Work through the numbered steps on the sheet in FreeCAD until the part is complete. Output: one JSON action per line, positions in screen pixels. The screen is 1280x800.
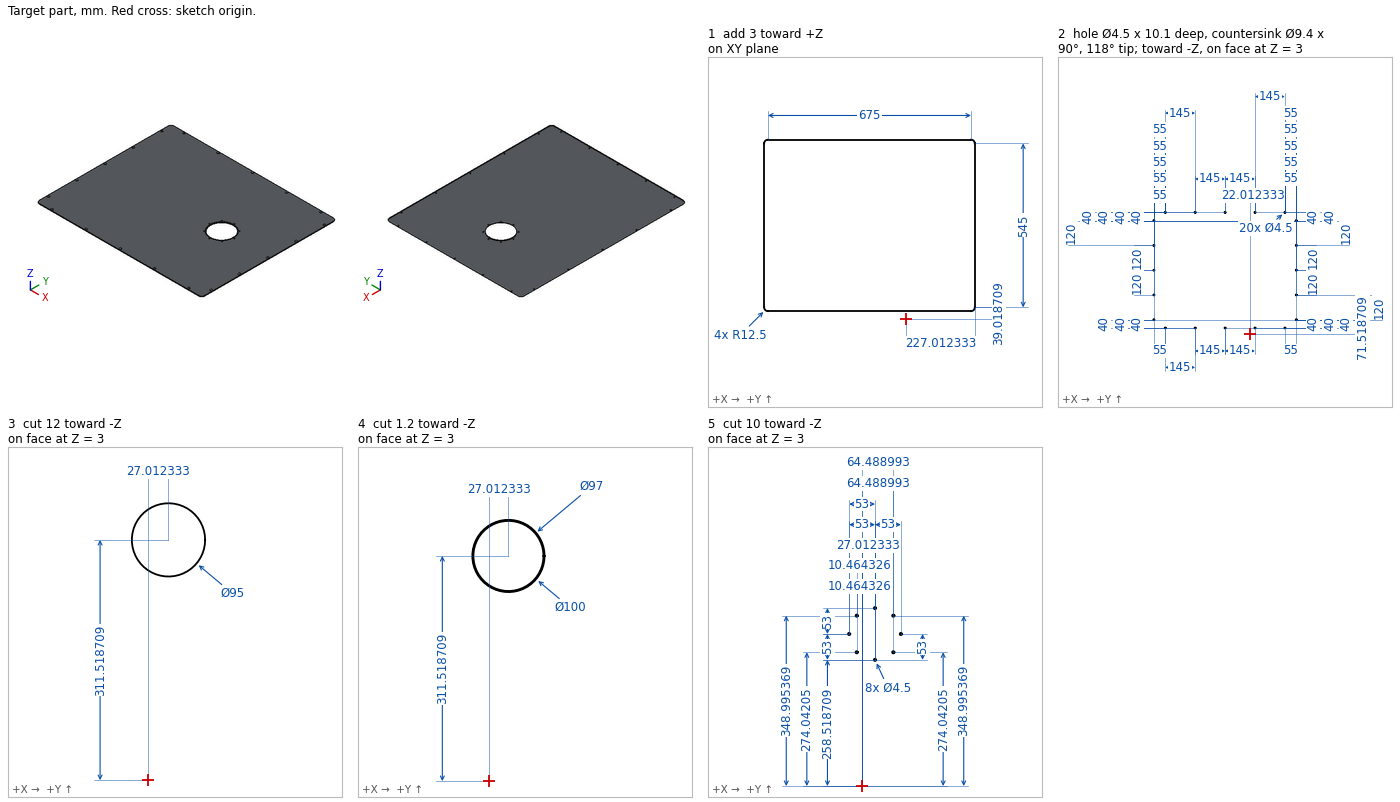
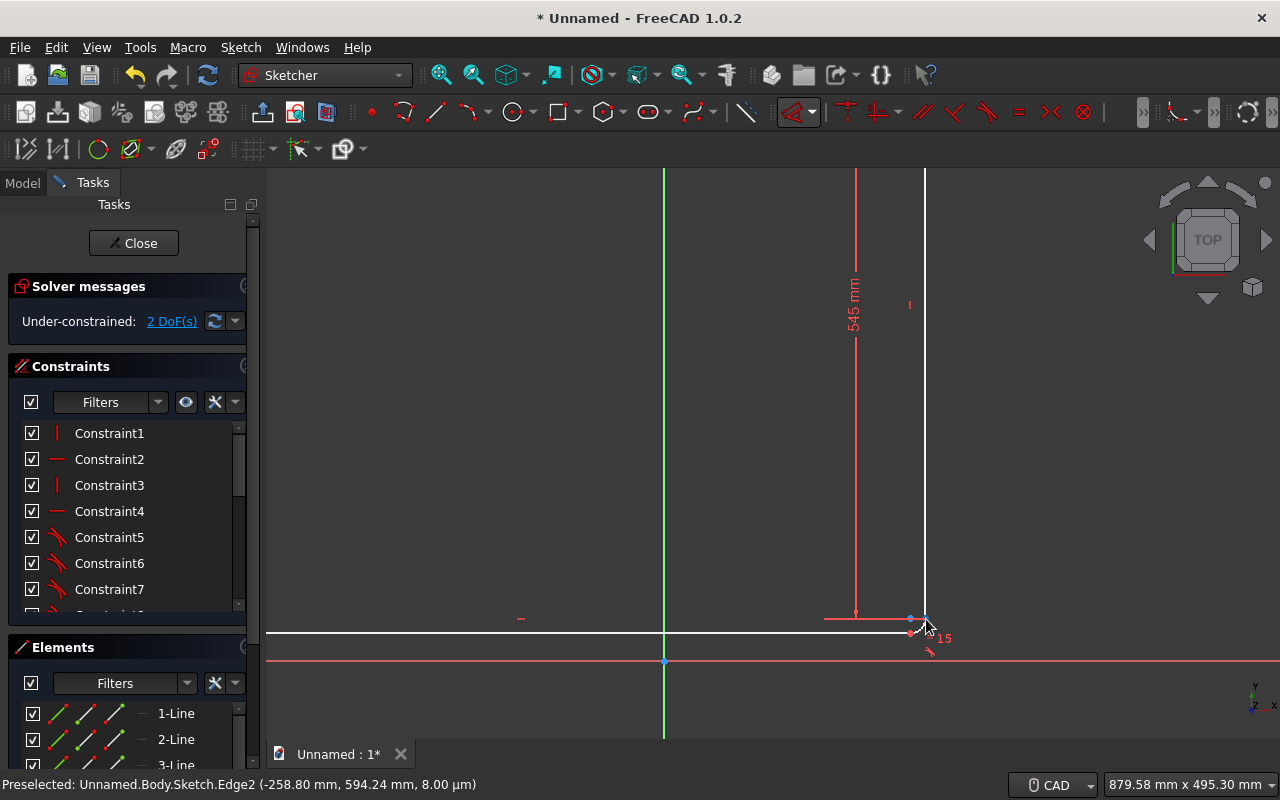
{"action": "left_click", "coordinate": [925, 619]}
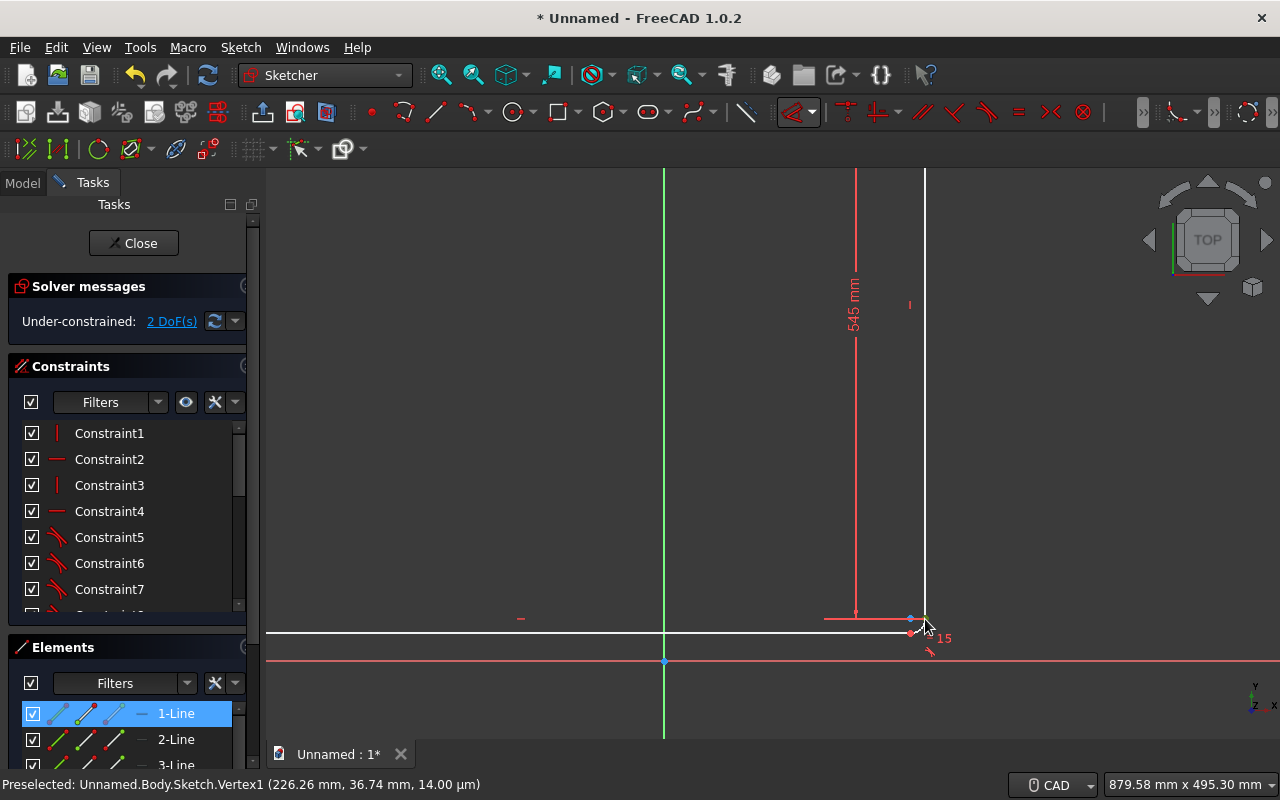
{"action": "left_click", "coordinate": [814, 112]}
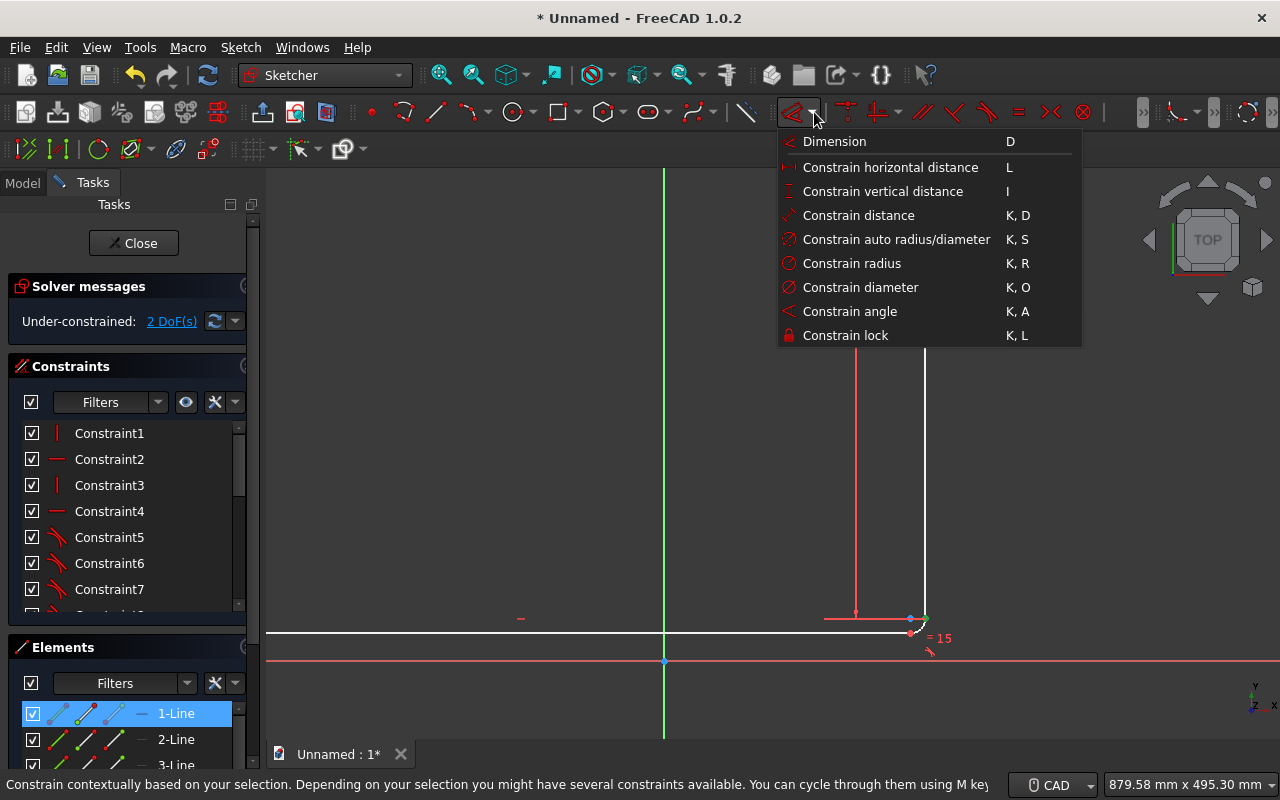
{"action": "left_click", "coordinate": [930, 191]}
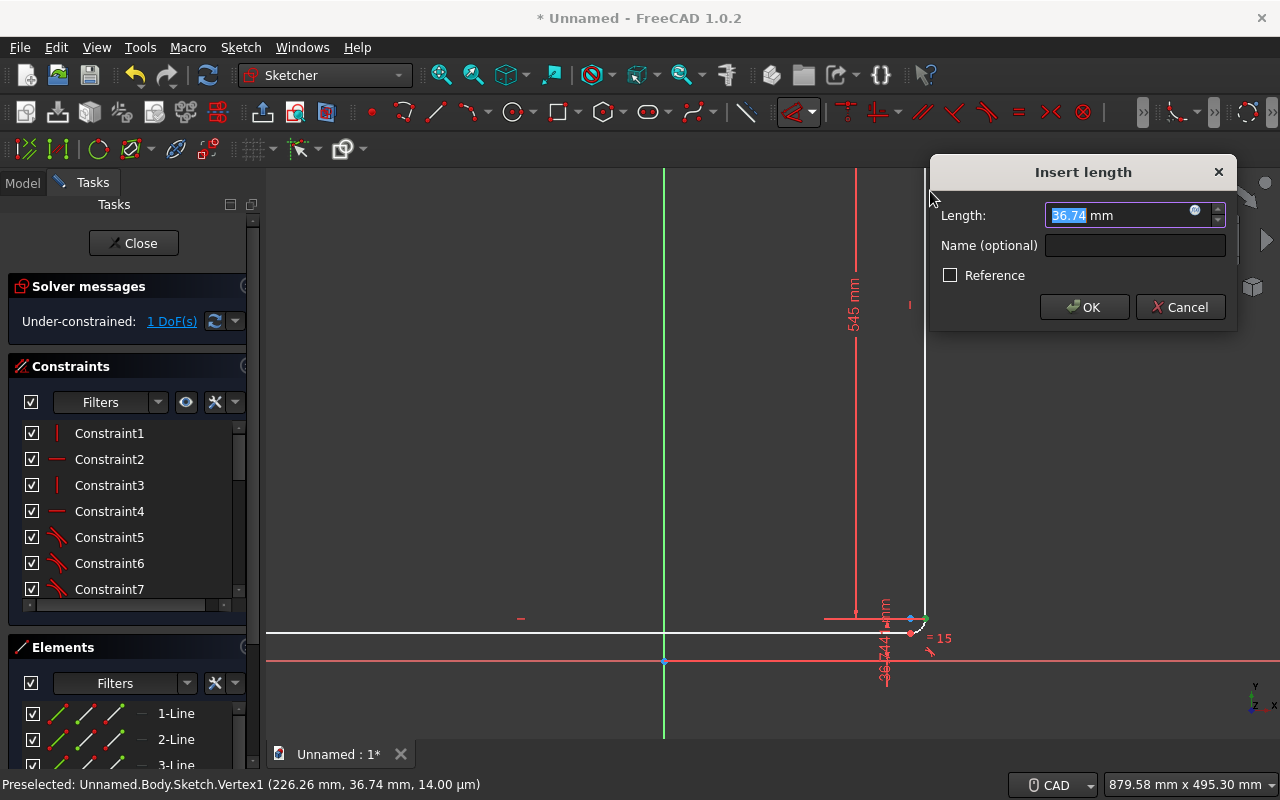
{"action": "type", "text": "39.018709"}
{"action": "key", "text": "Return"}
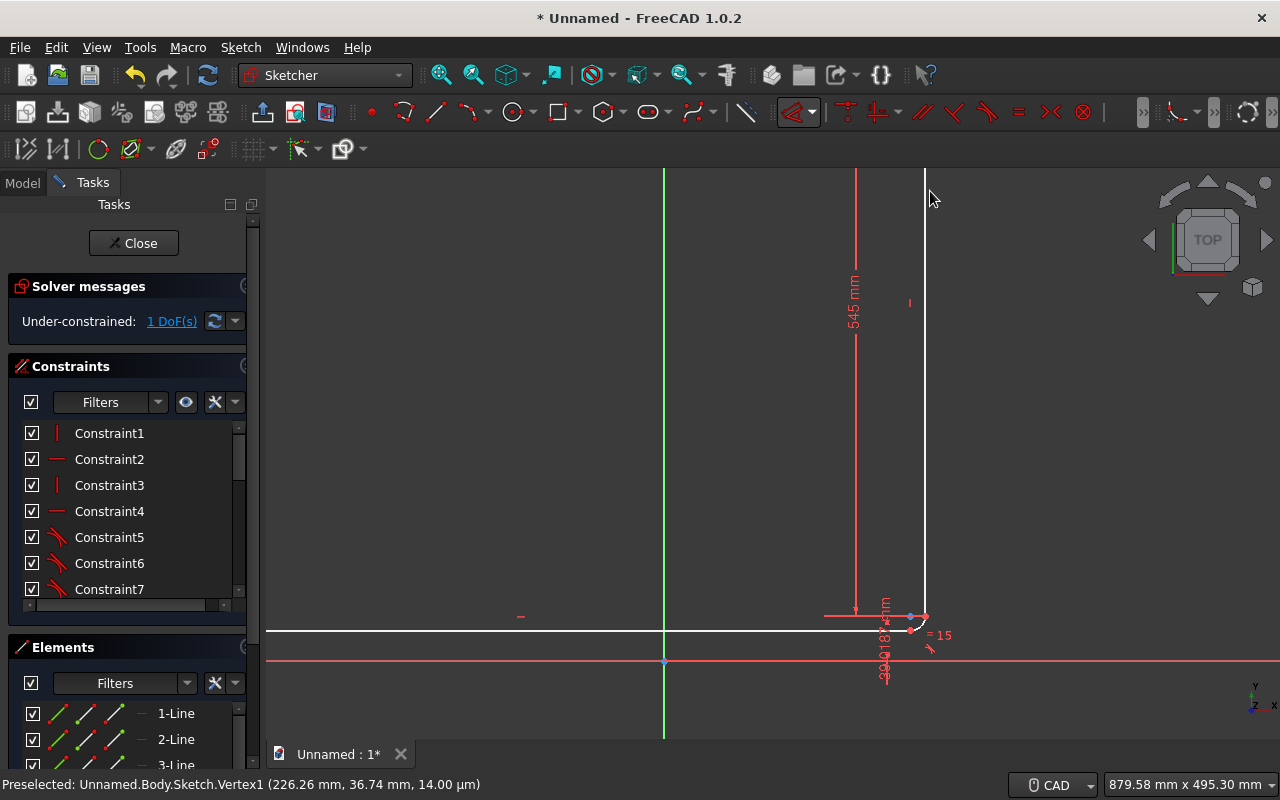
{"action": "left_click", "coordinate": [925, 616]}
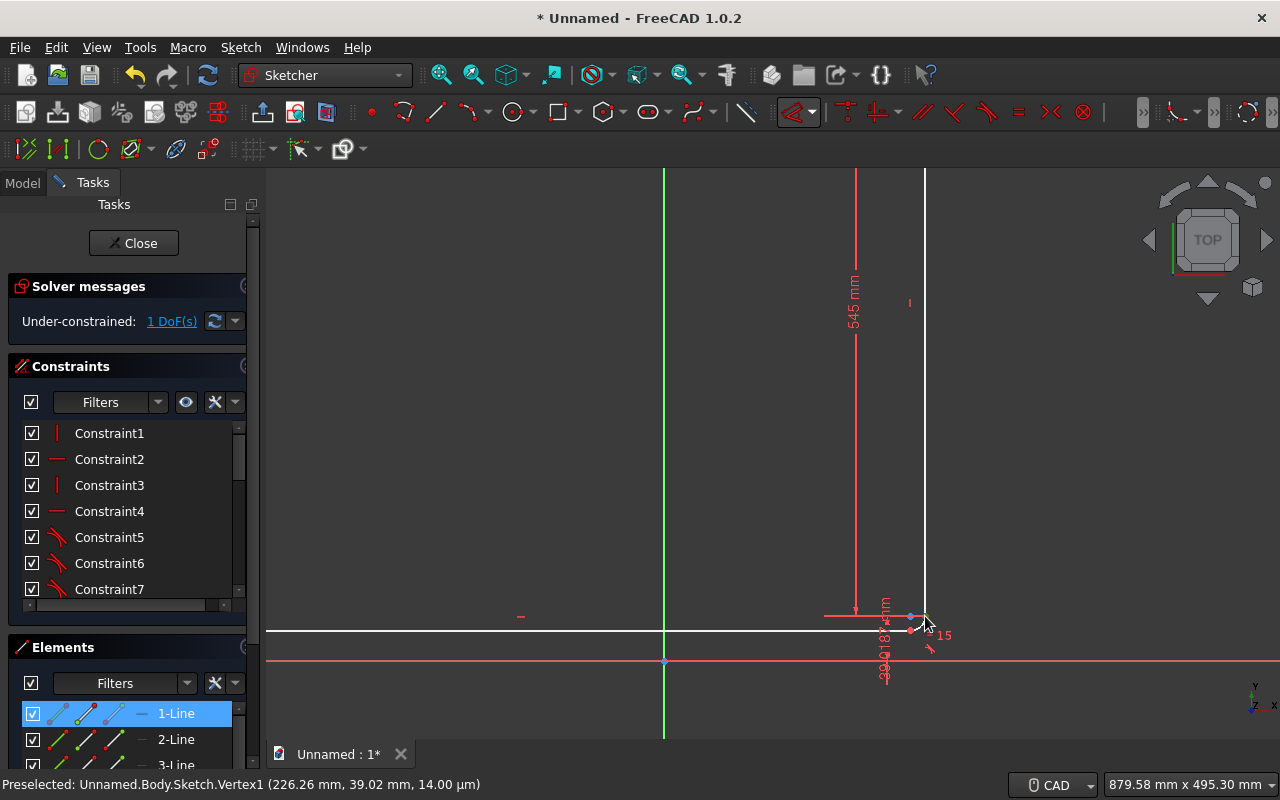
{"action": "key", "text": "l"}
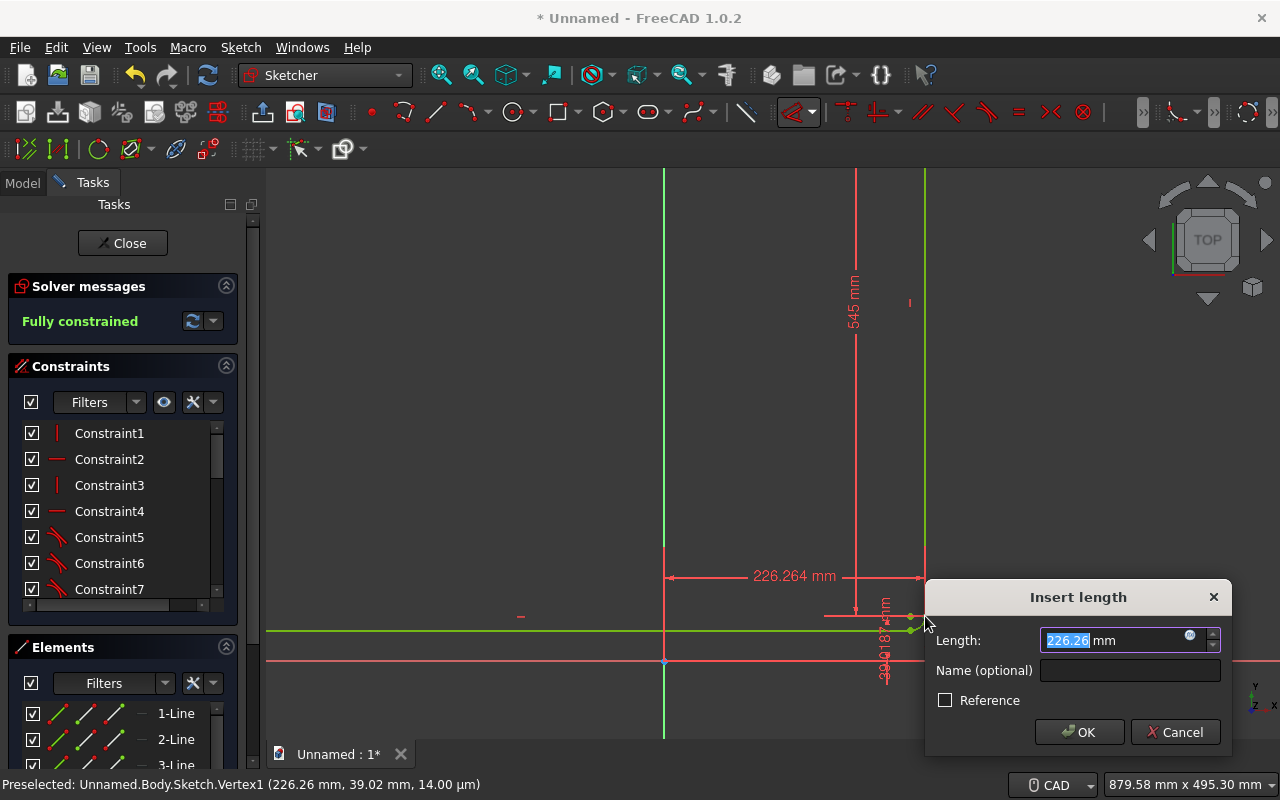
{"action": "type", "text": "227.012333"}
{"action": "key", "text": "Return"}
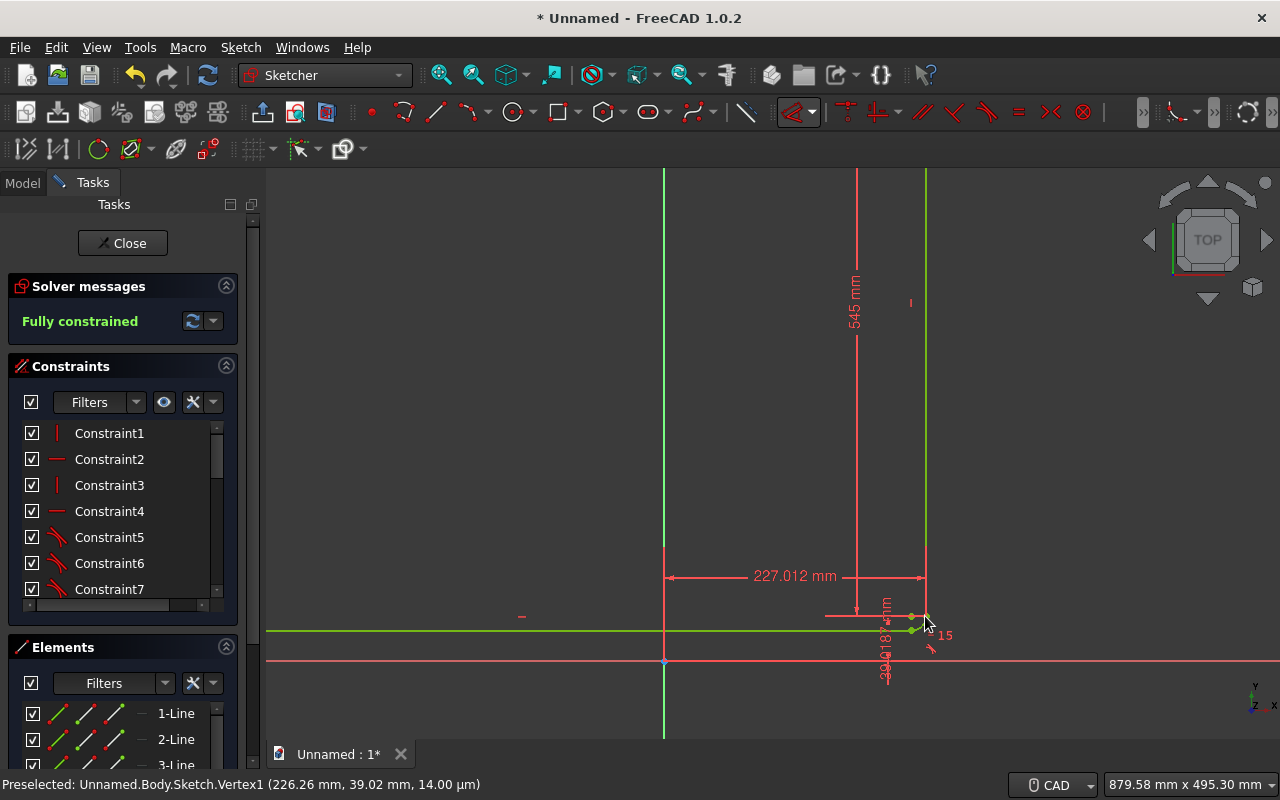
{"action": "left_click", "coordinate": [123, 243]}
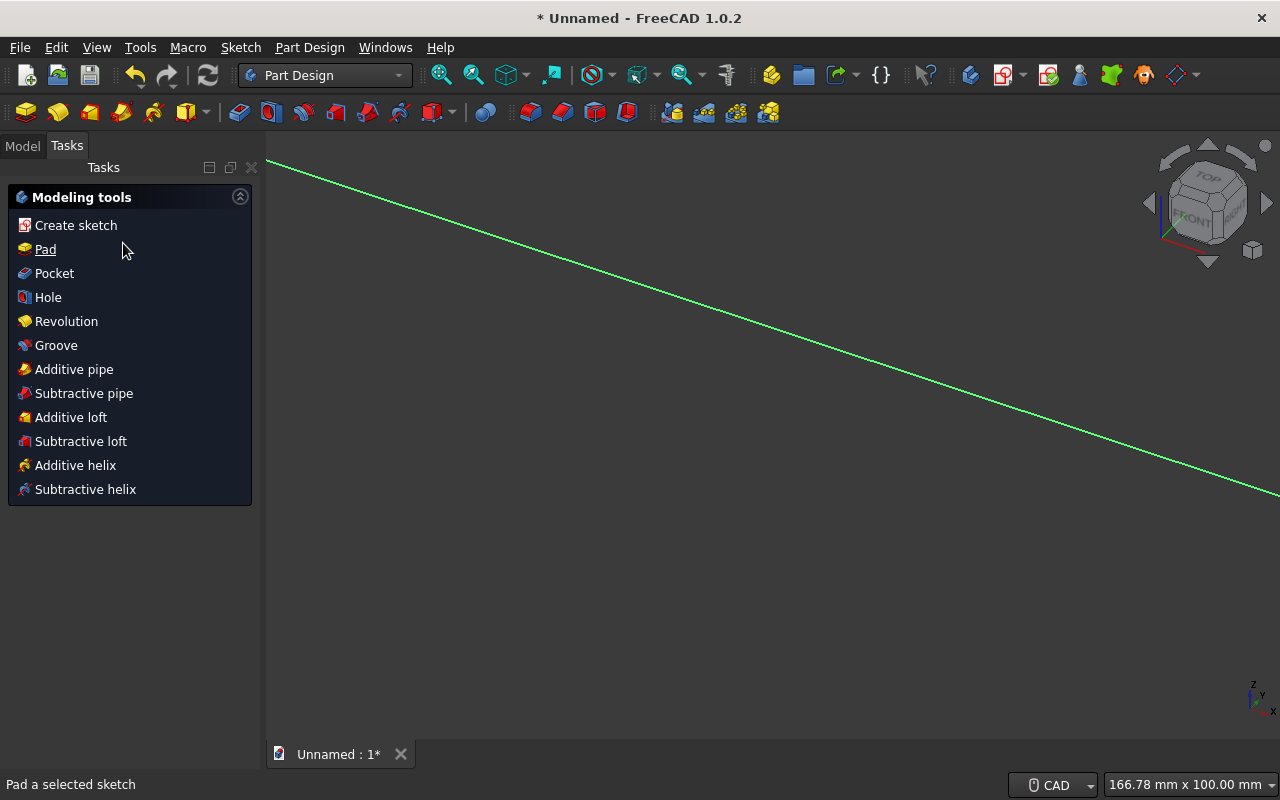
{"action": "left_click", "coordinate": [26, 112]}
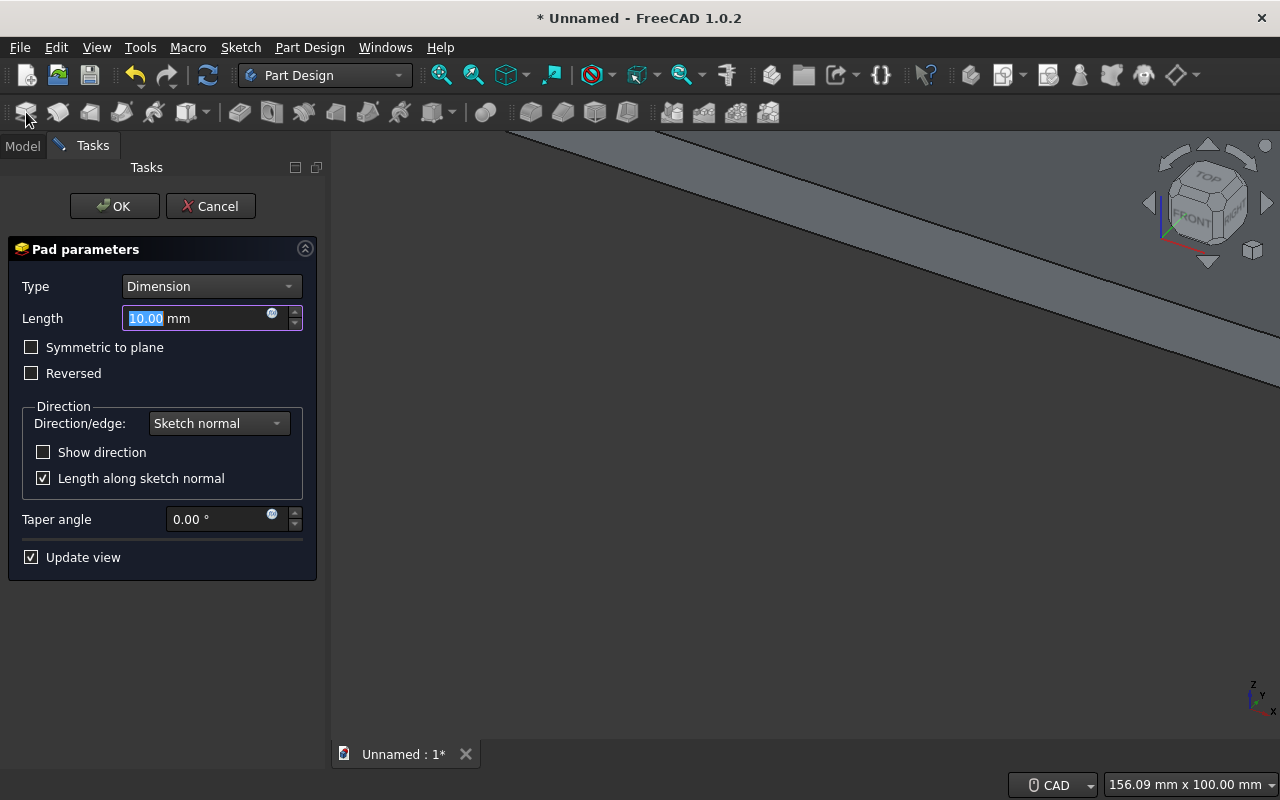
{"action": "type", "text": "3"}
{"action": "key", "text": "Tab"}